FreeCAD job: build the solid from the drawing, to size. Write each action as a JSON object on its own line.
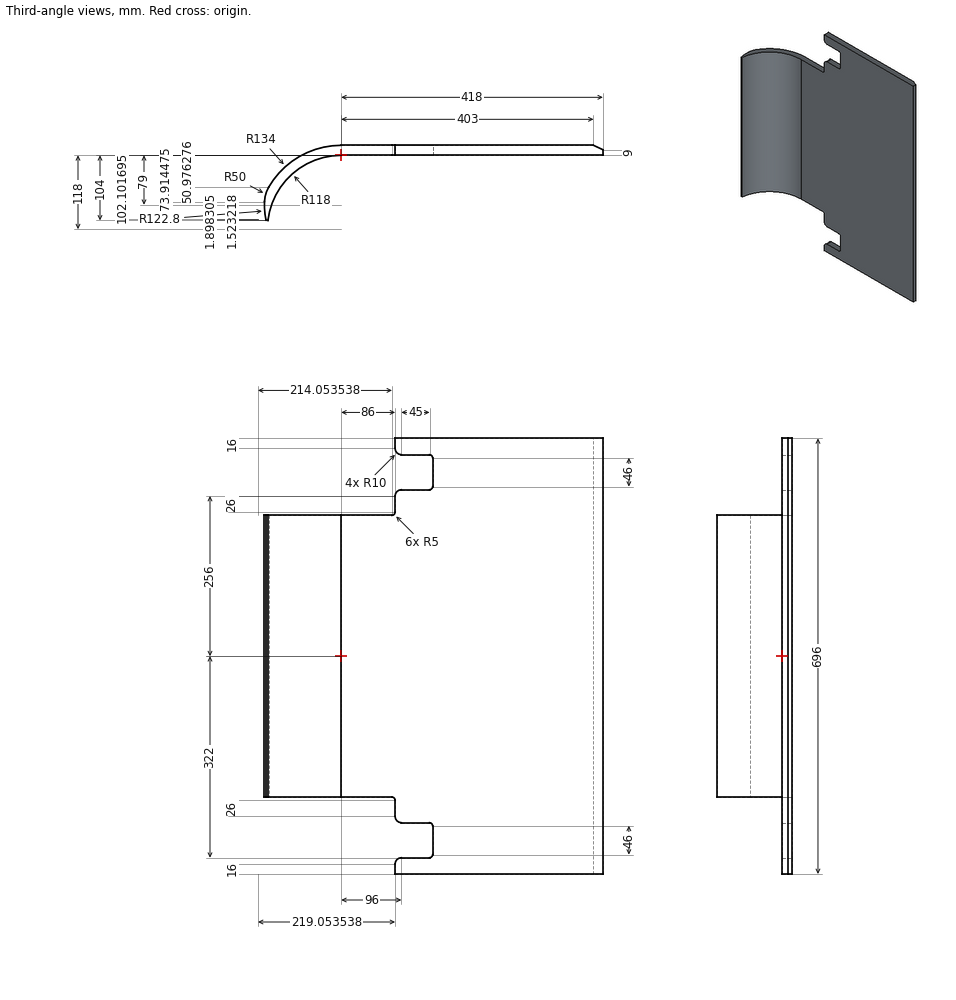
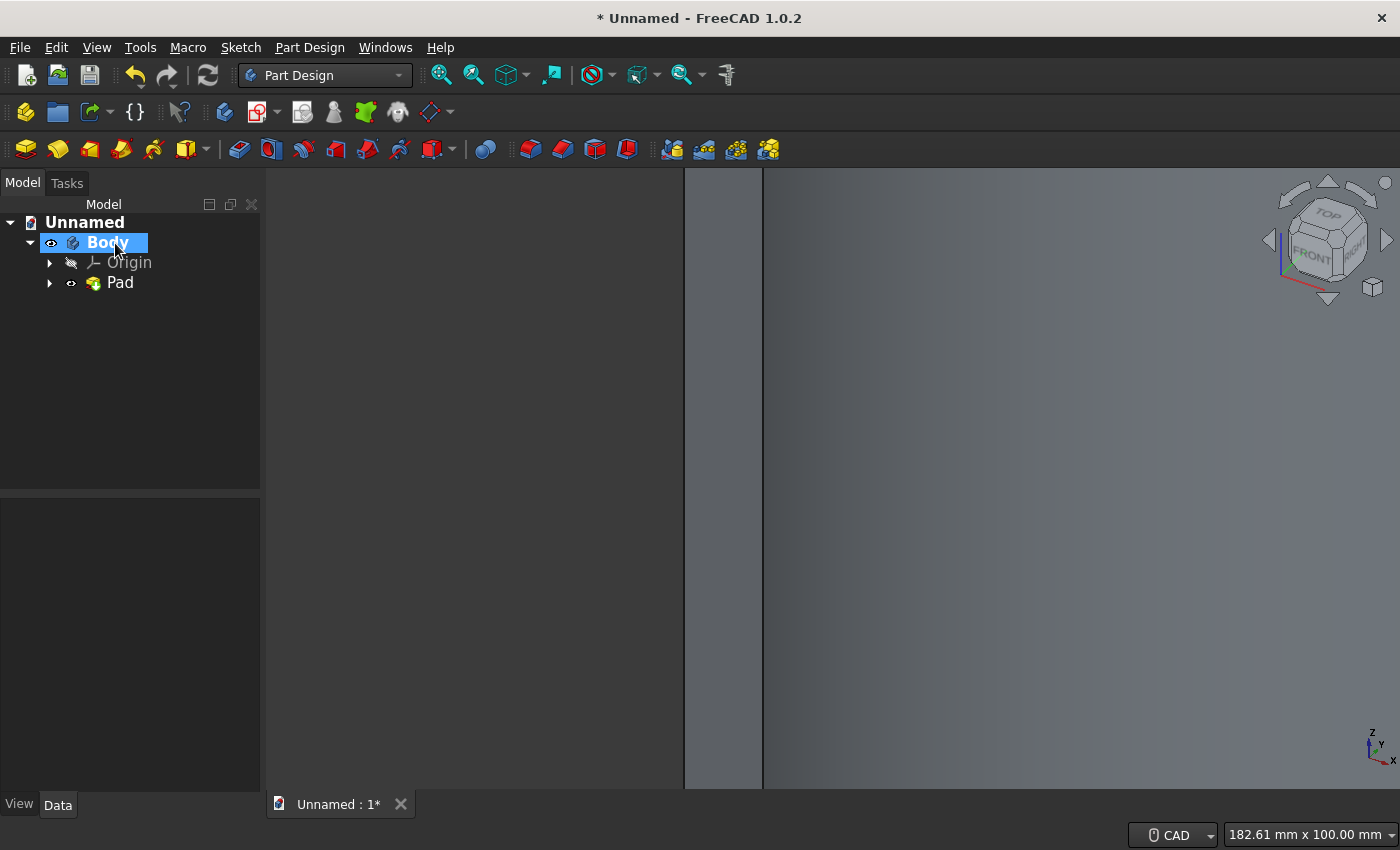
{"action": "left_click", "coordinate": [442, 76]}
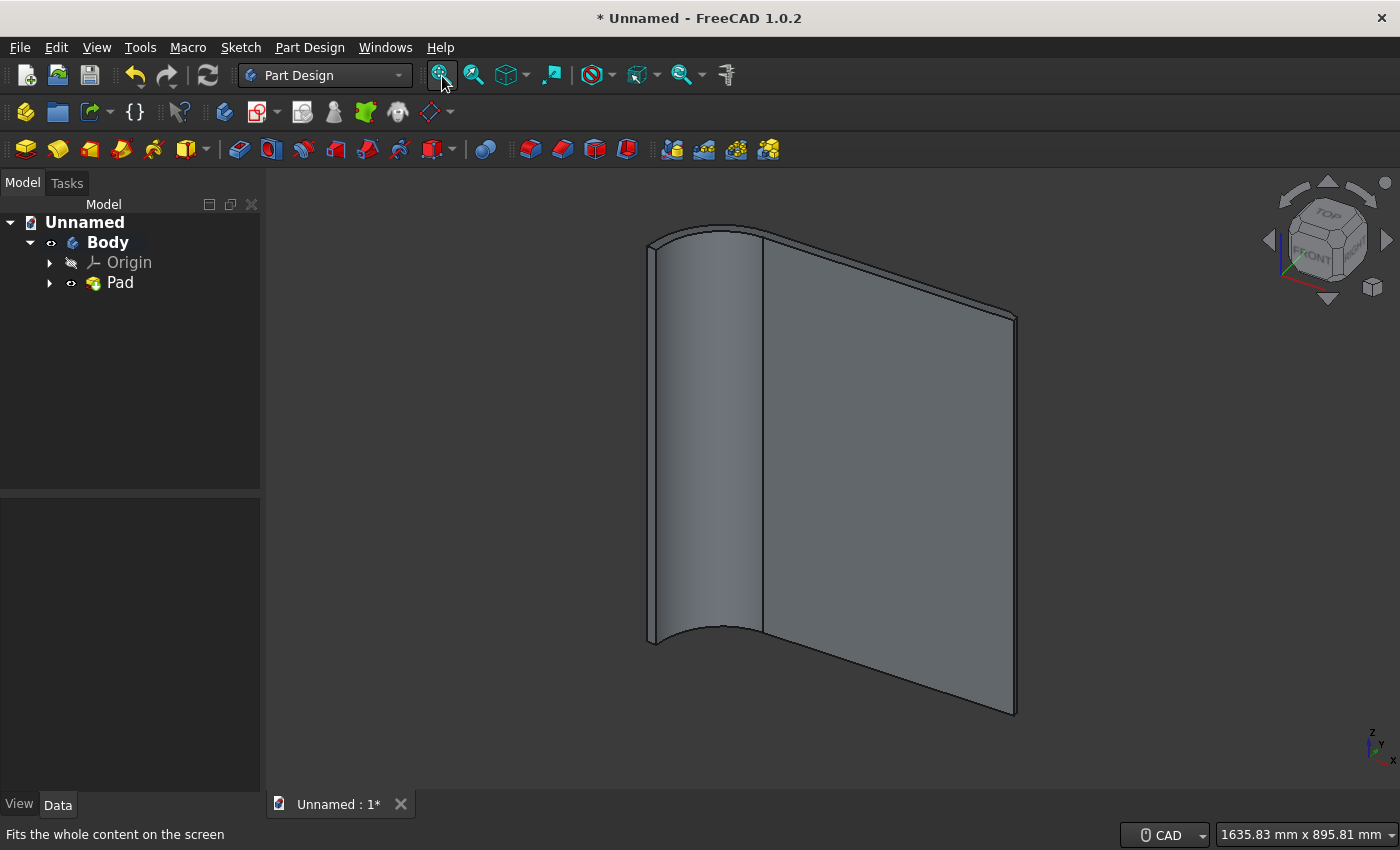
{"action": "left_click", "coordinate": [258, 112]}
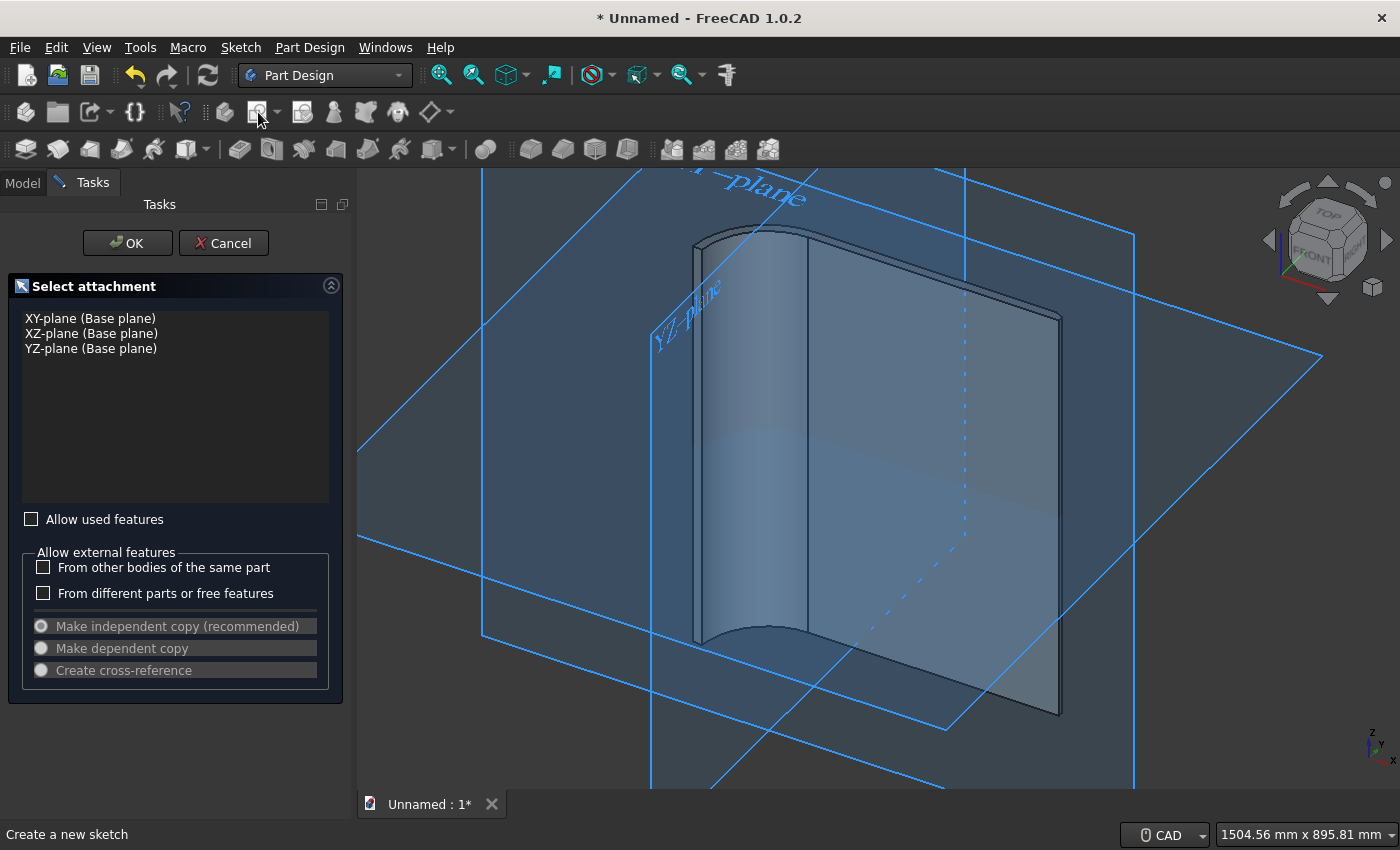
{"action": "left_click", "coordinate": [82, 334]}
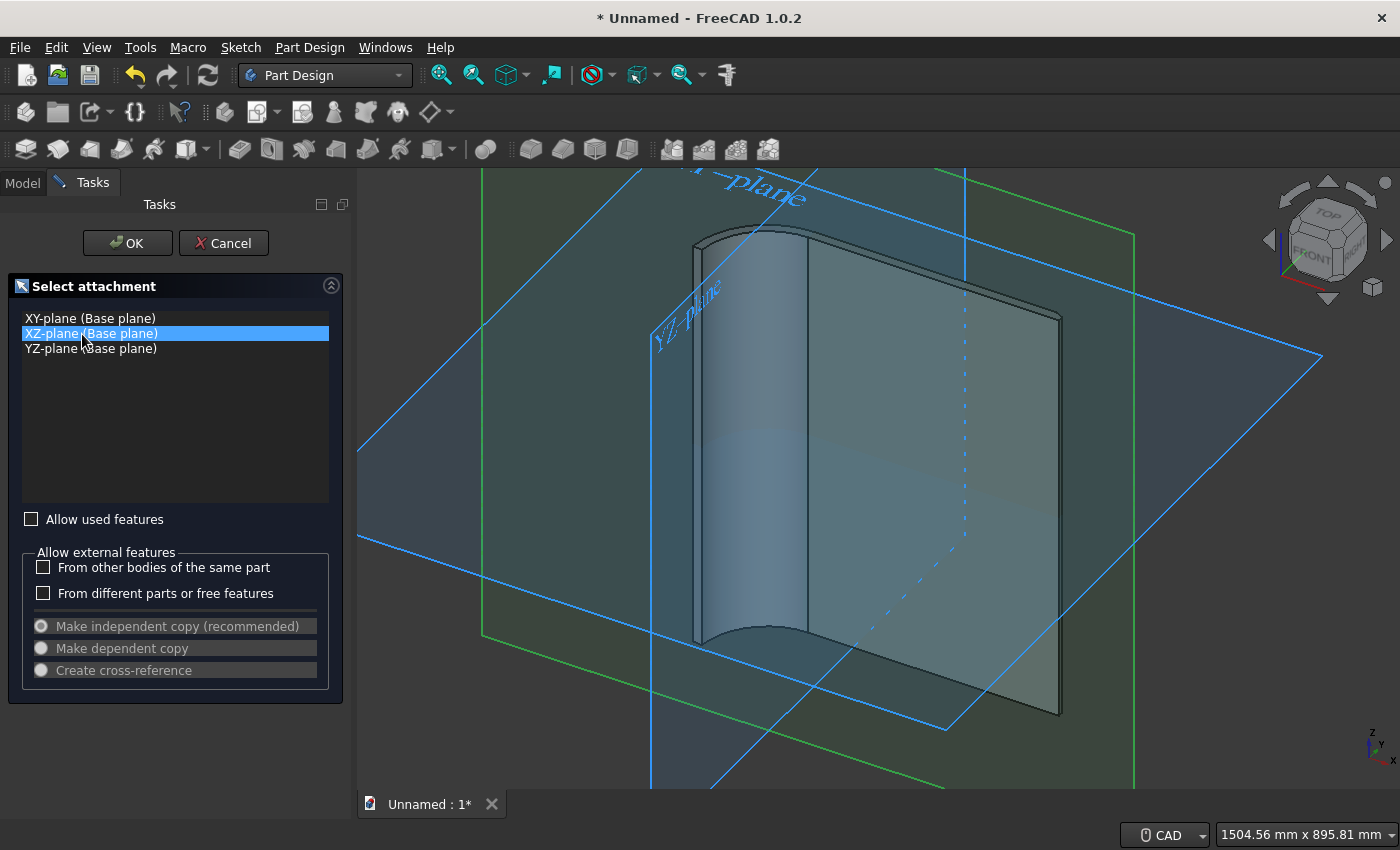
{"action": "left_click", "coordinate": [128, 243]}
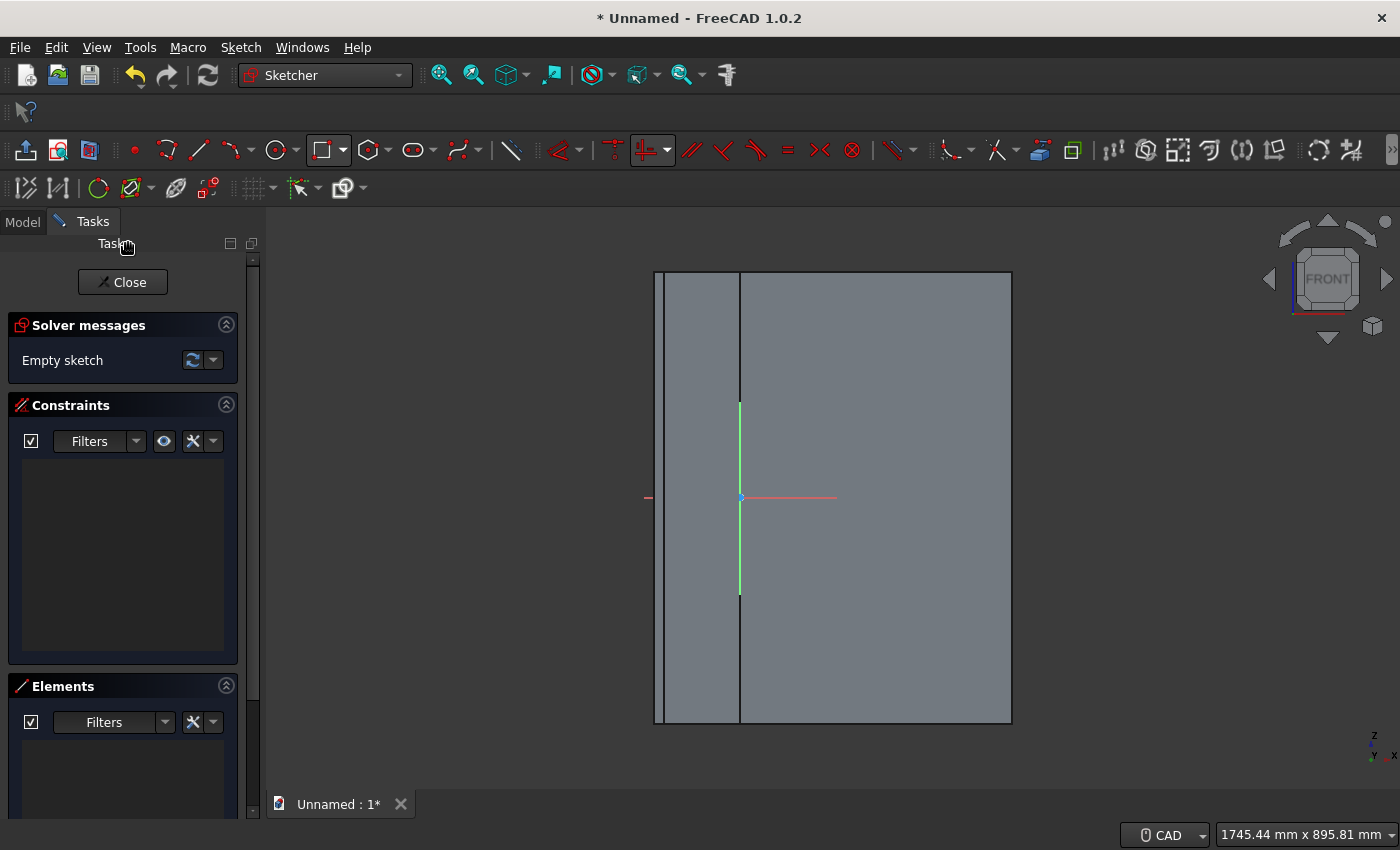
{"action": "left_click", "coordinate": [90, 150]}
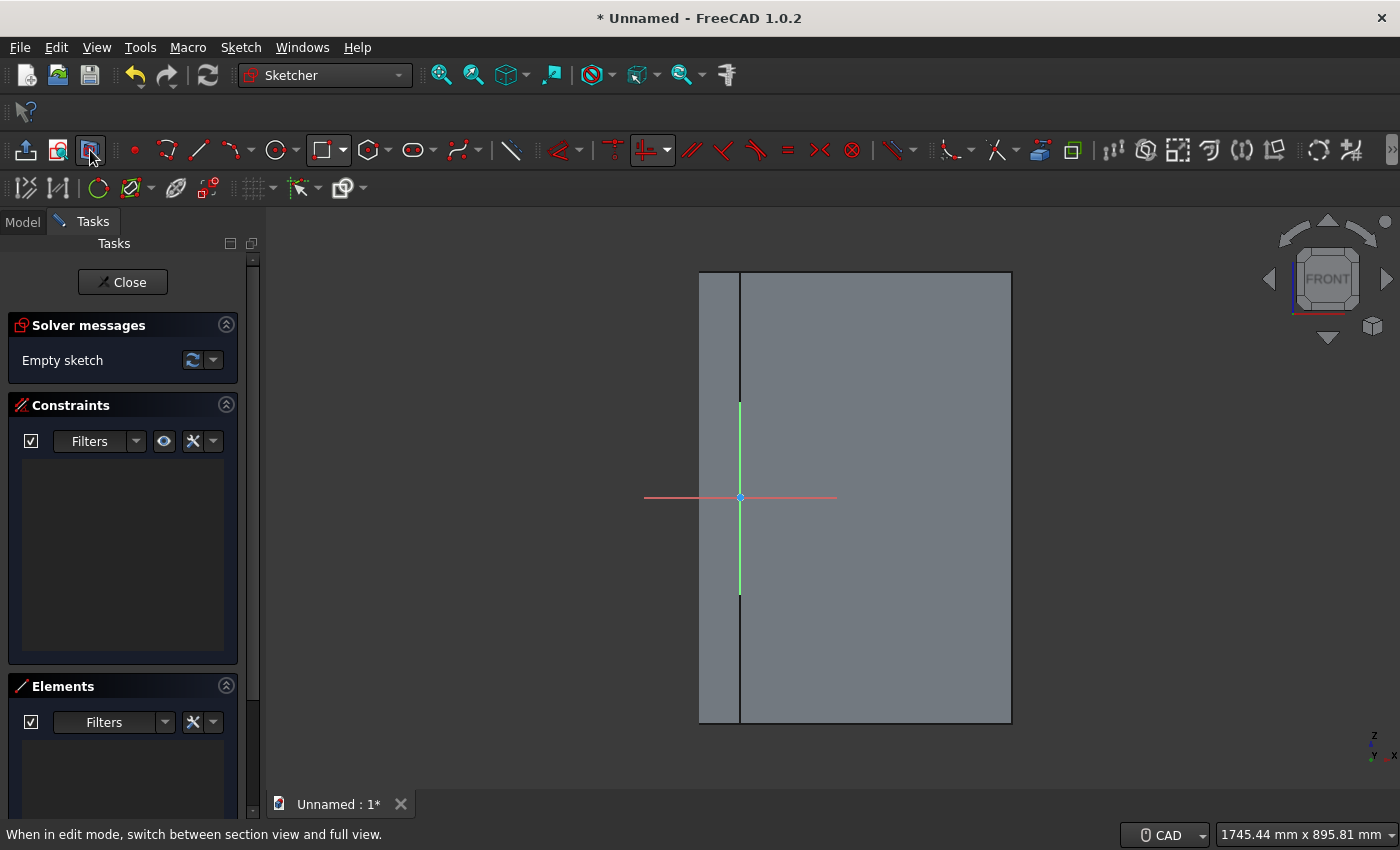
{"action": "left_click", "coordinate": [200, 150]}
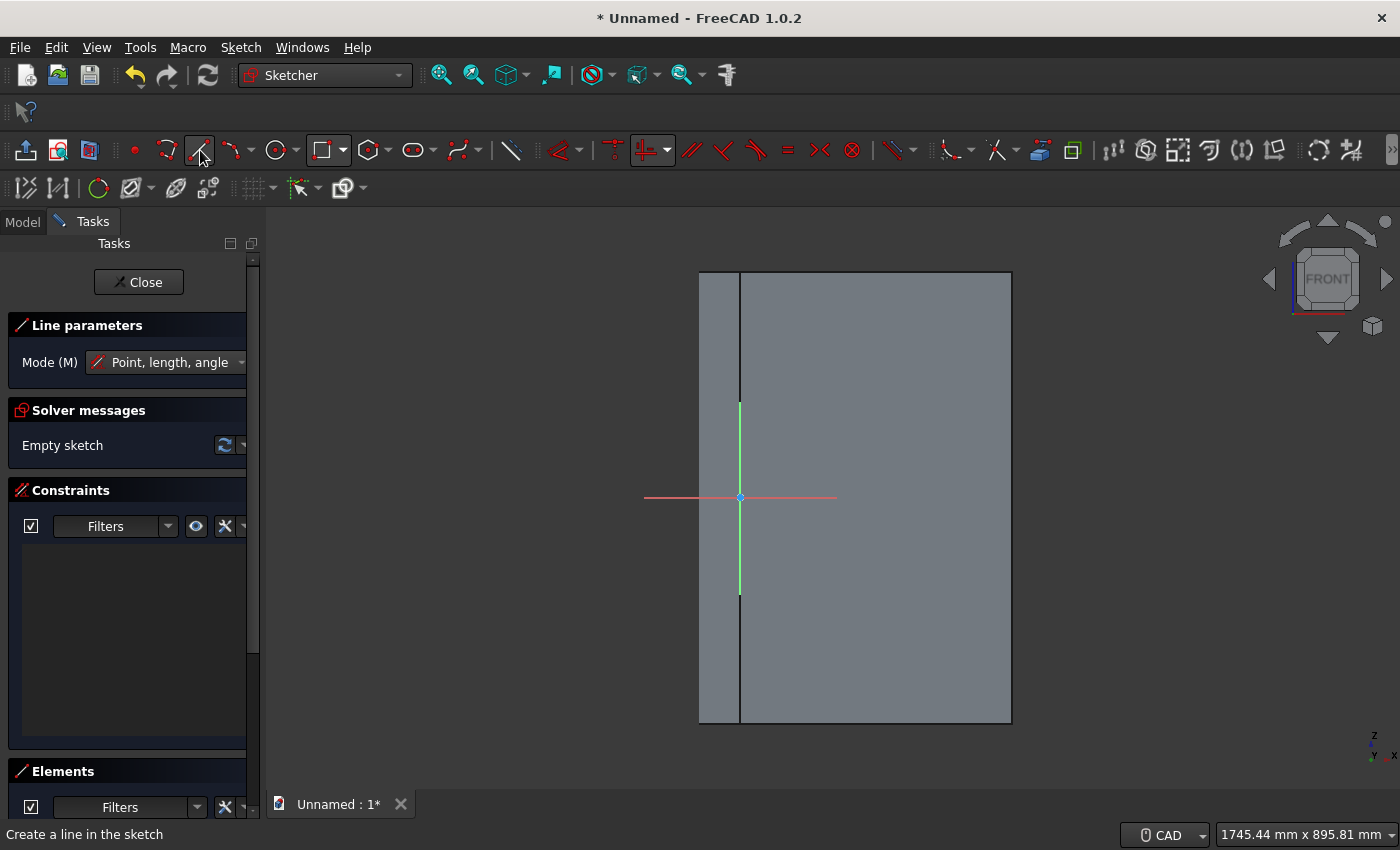
{"action": "left_click", "coordinate": [796, 332]}
{"action": "left_click", "coordinate": [796, 349]}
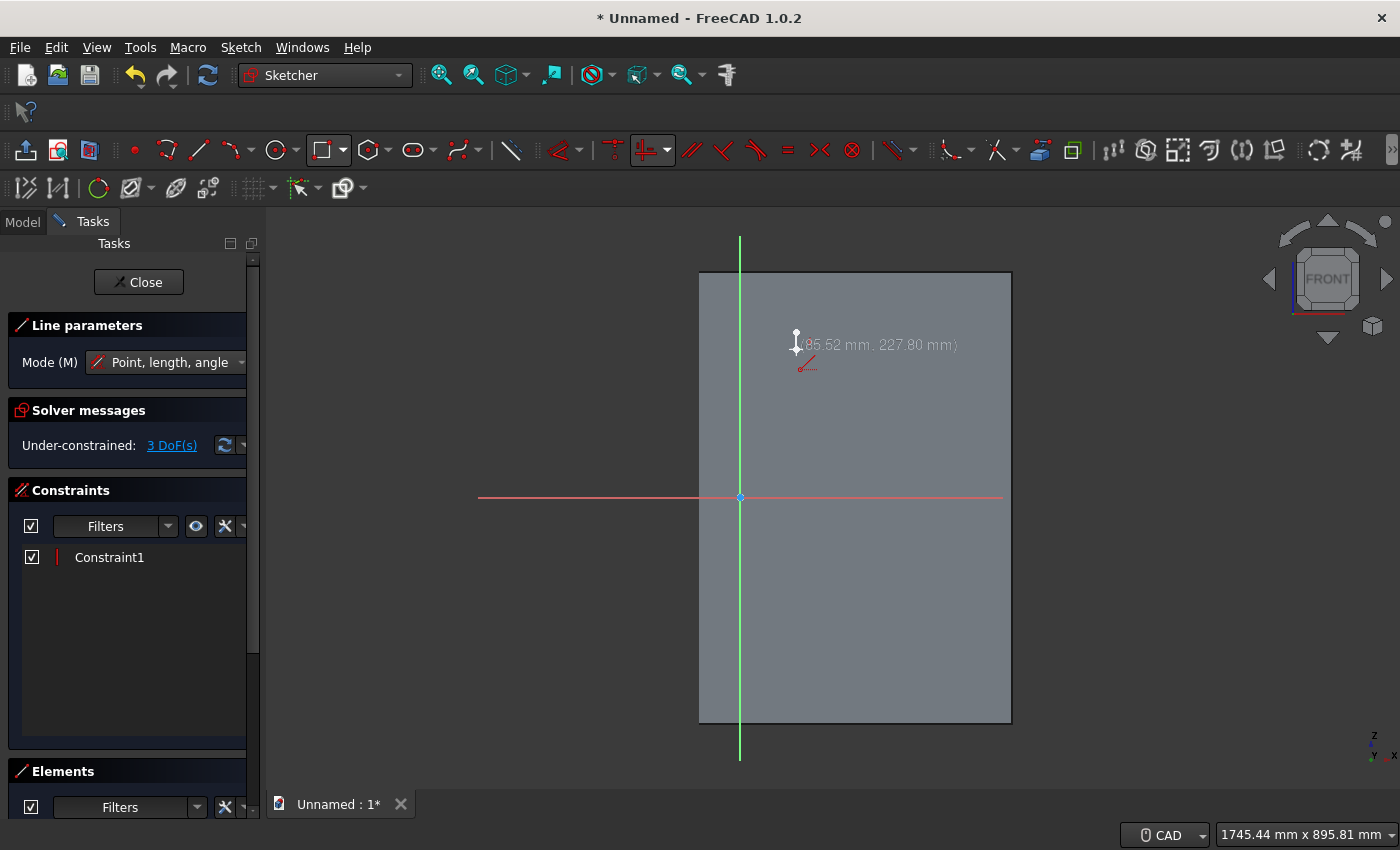
{"action": "left_click", "coordinate": [168, 150]}